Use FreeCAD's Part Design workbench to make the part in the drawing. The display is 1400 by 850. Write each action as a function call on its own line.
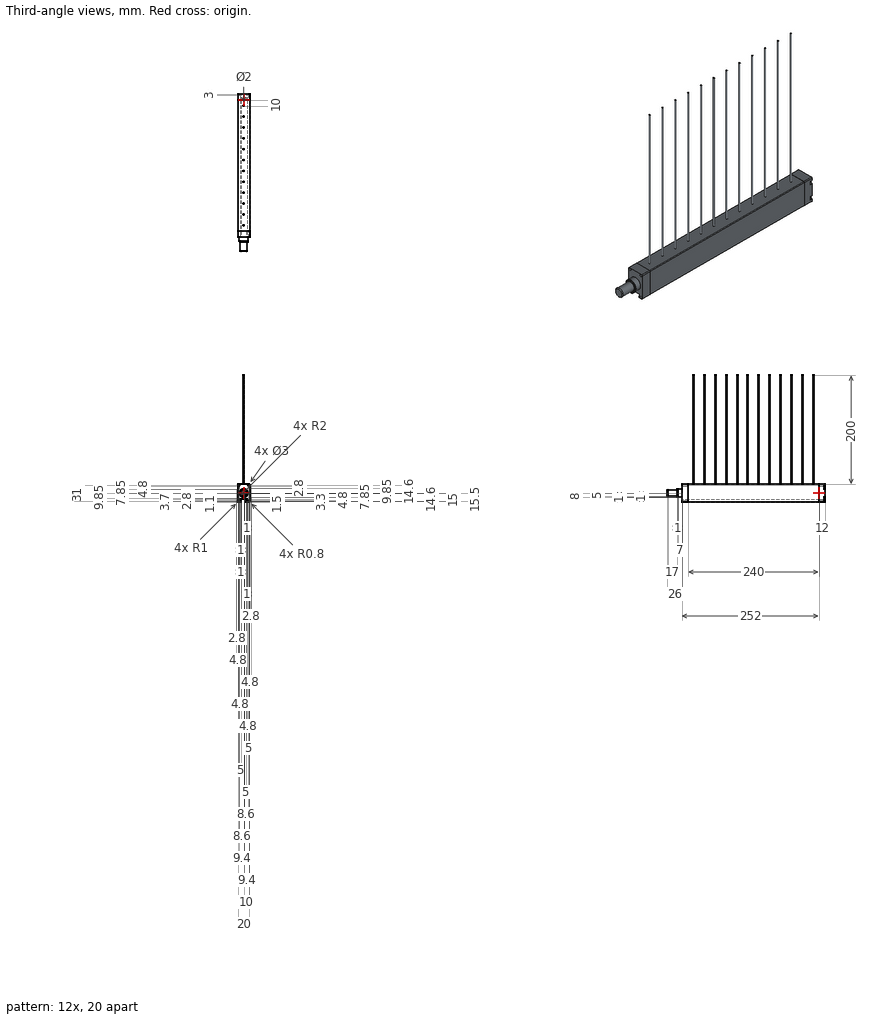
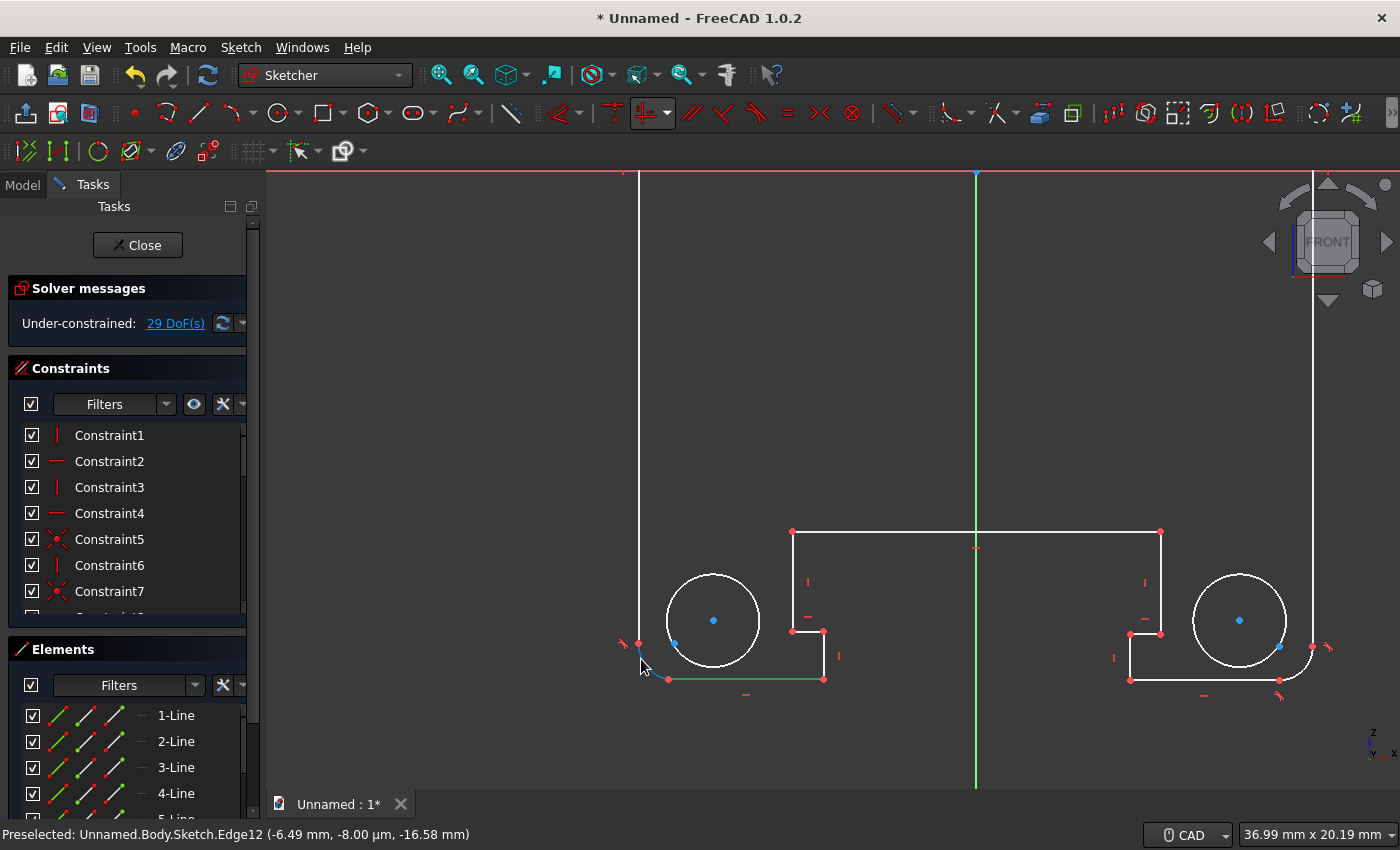
click(642, 659)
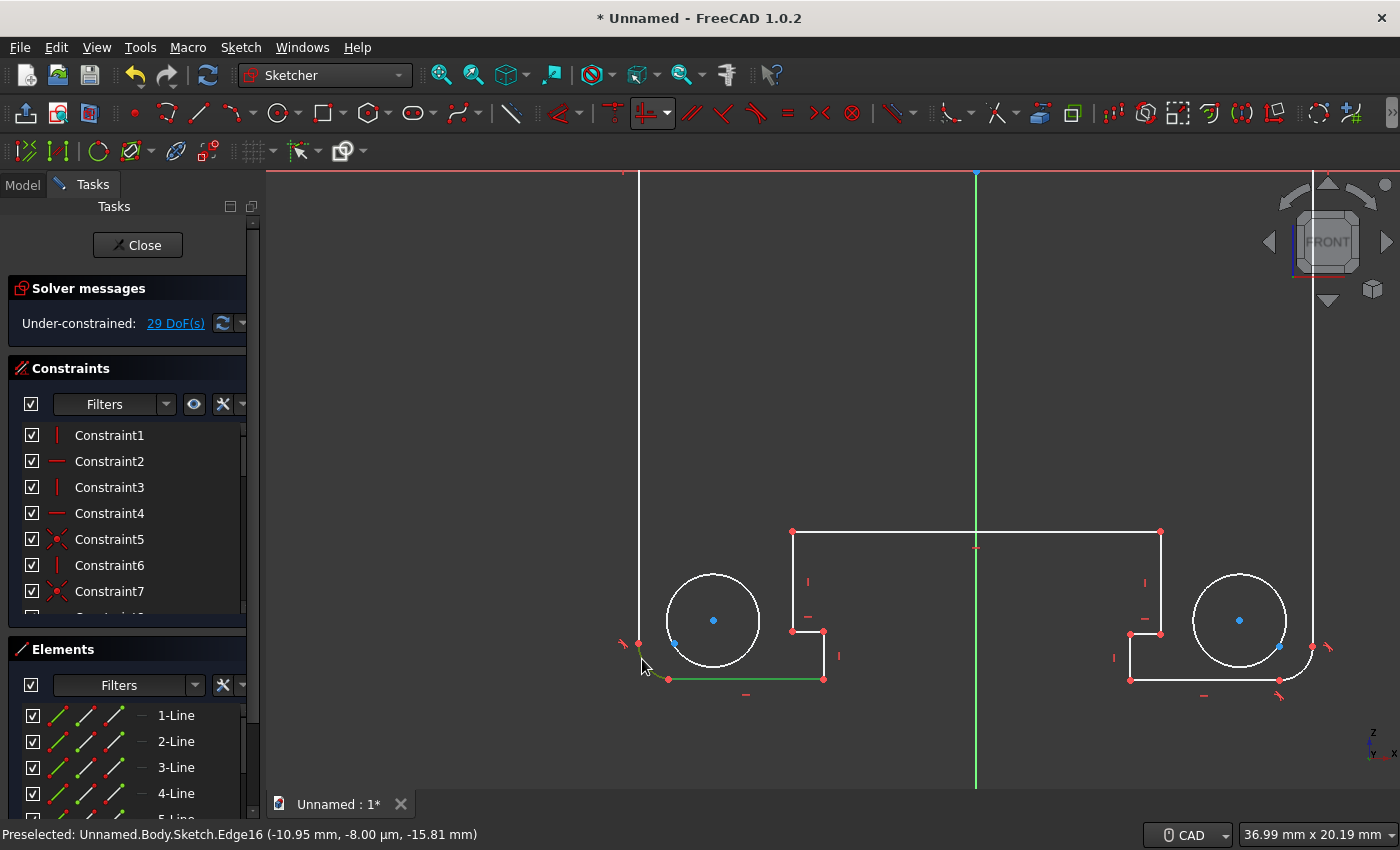
click(756, 114)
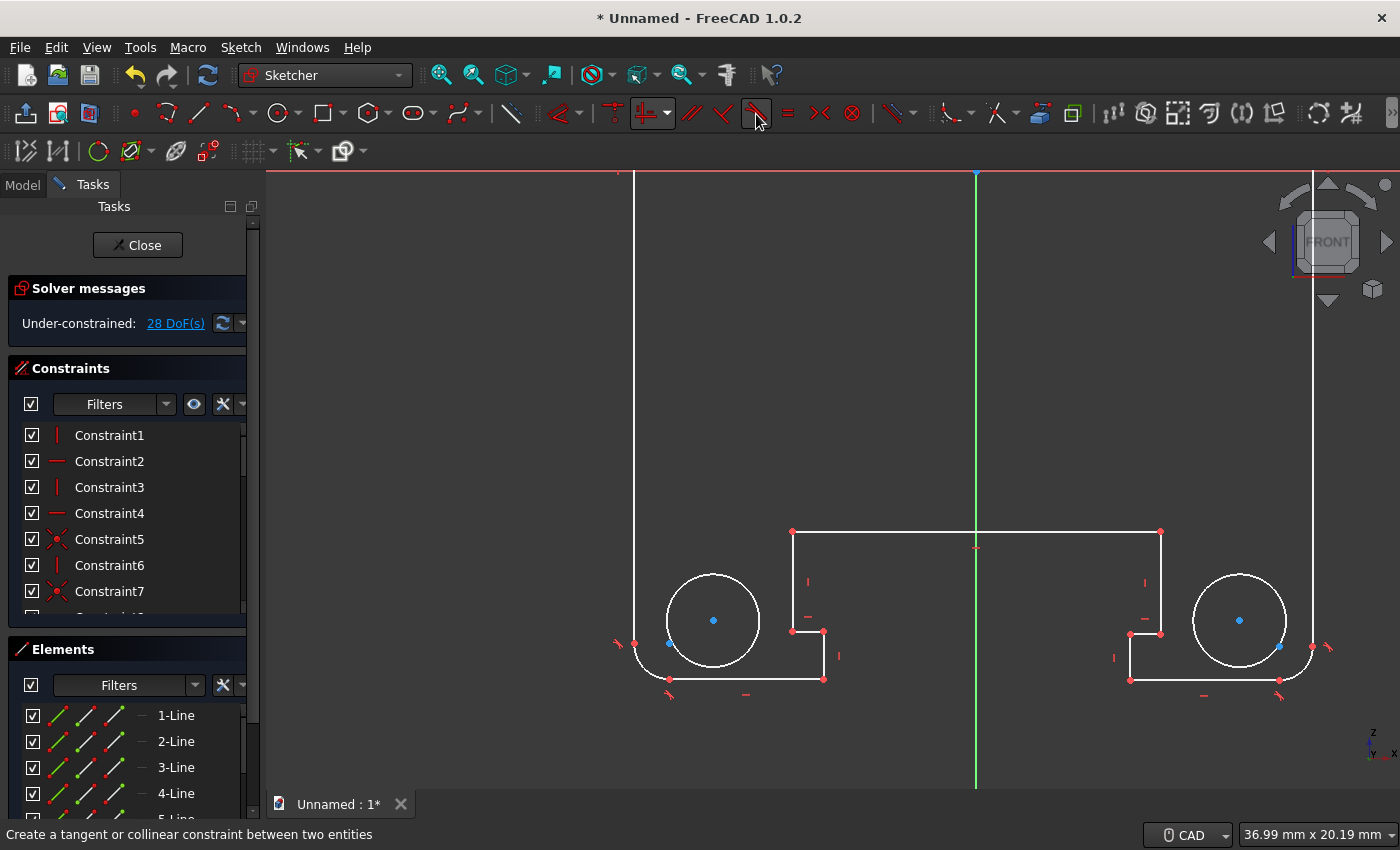
scroll(641, 659, down, 5)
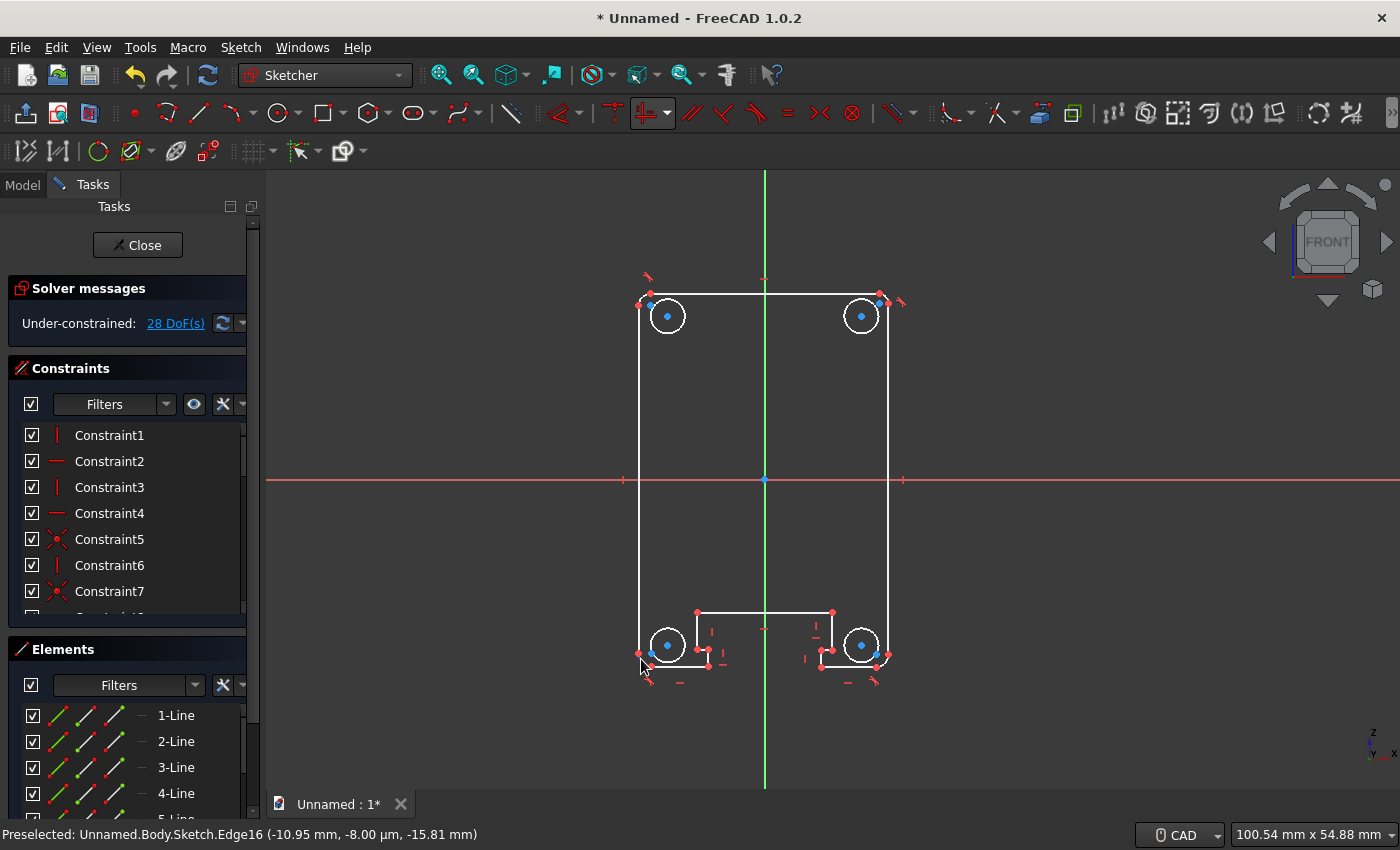
scroll(645, 295, up, 5)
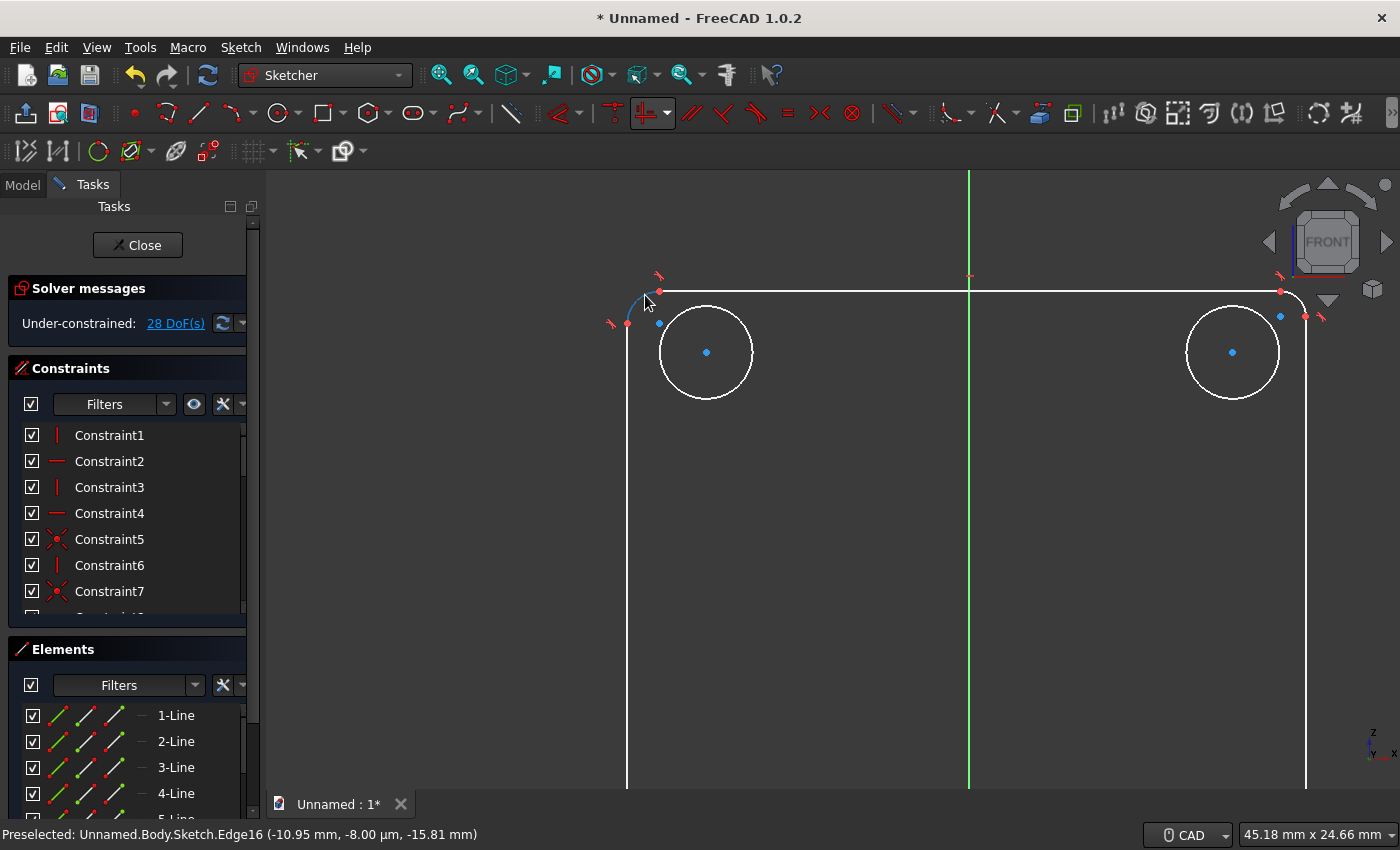
click(645, 295)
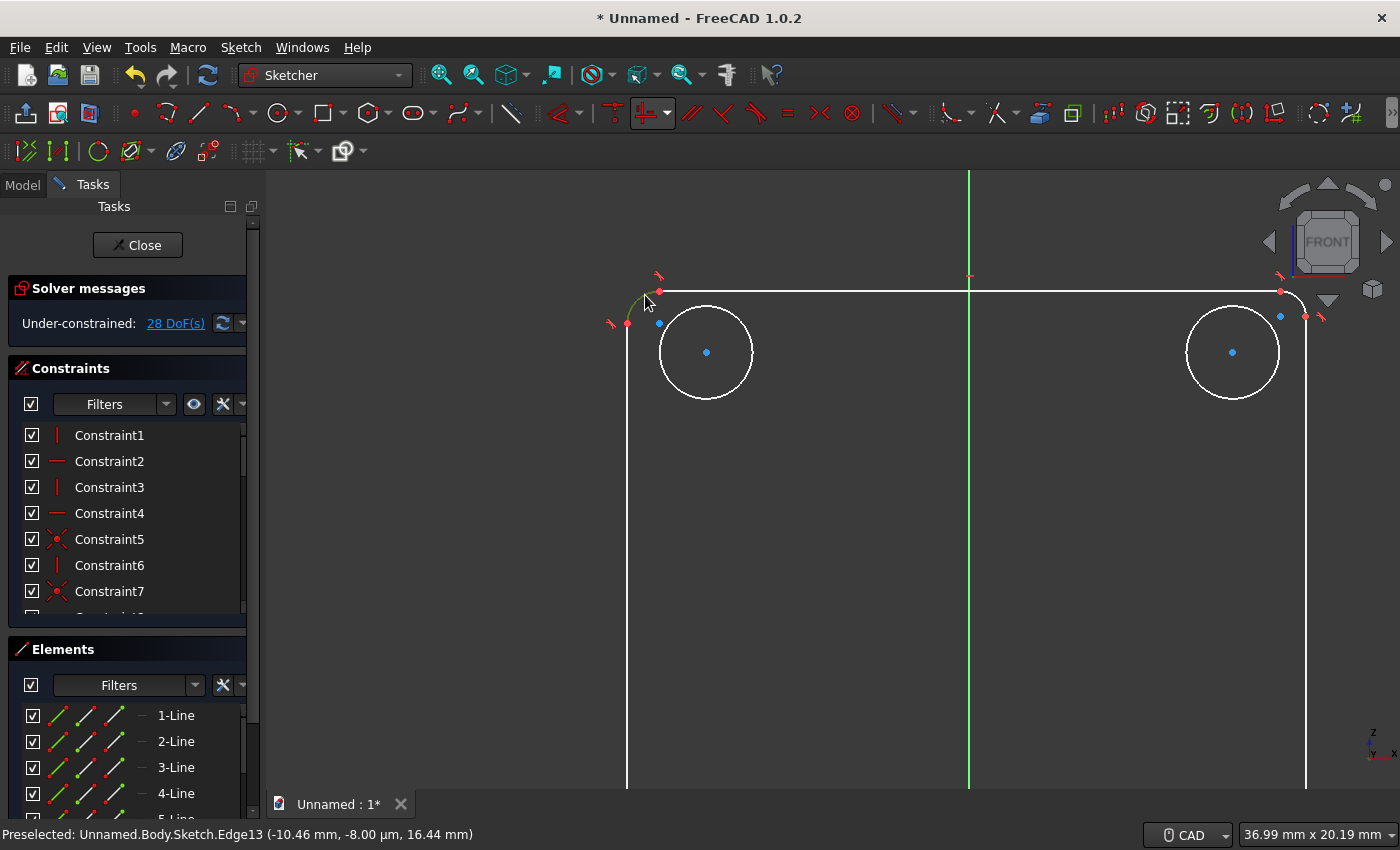
scroll(645, 294, down, 5)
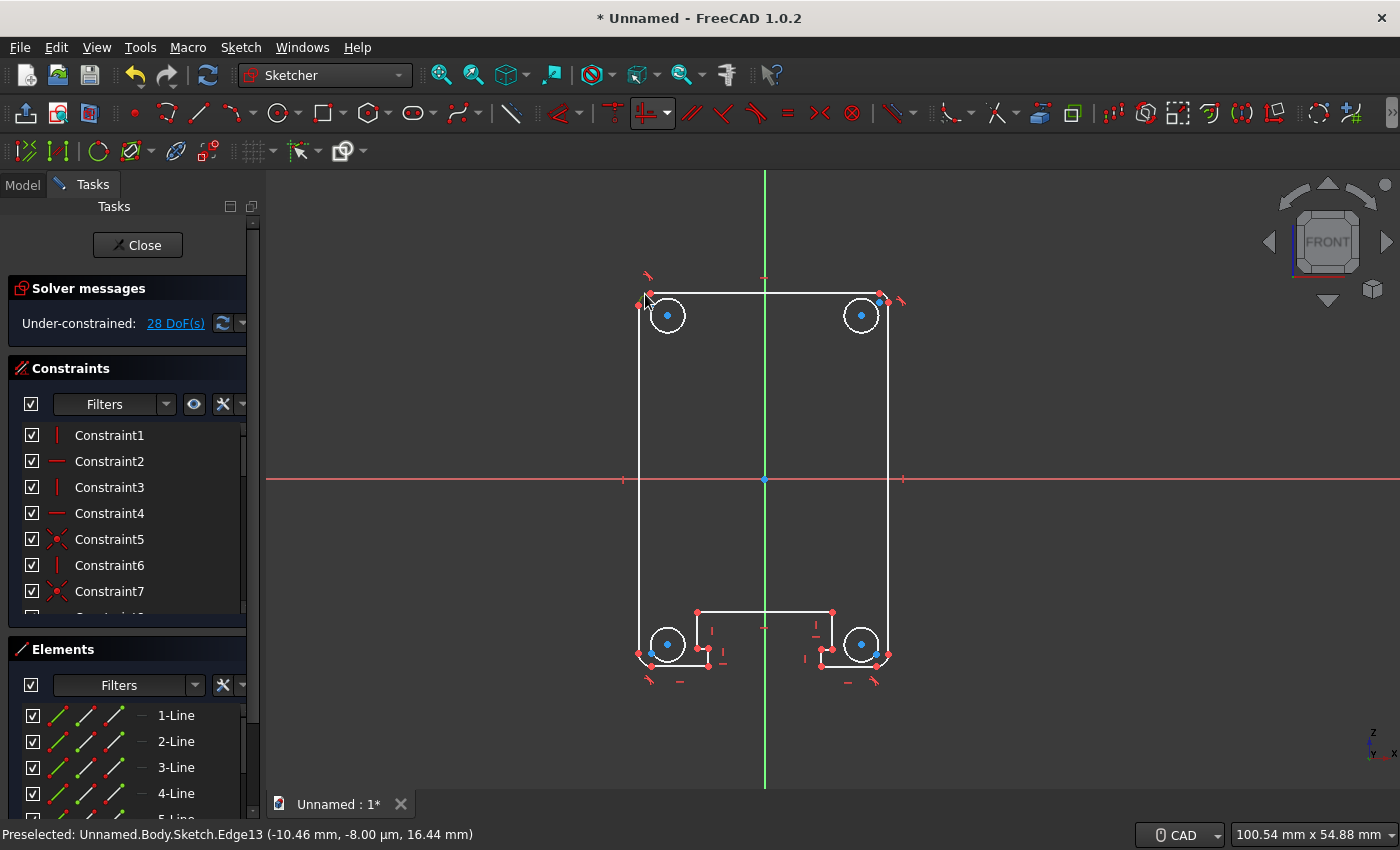
scroll(887, 298, up, 6)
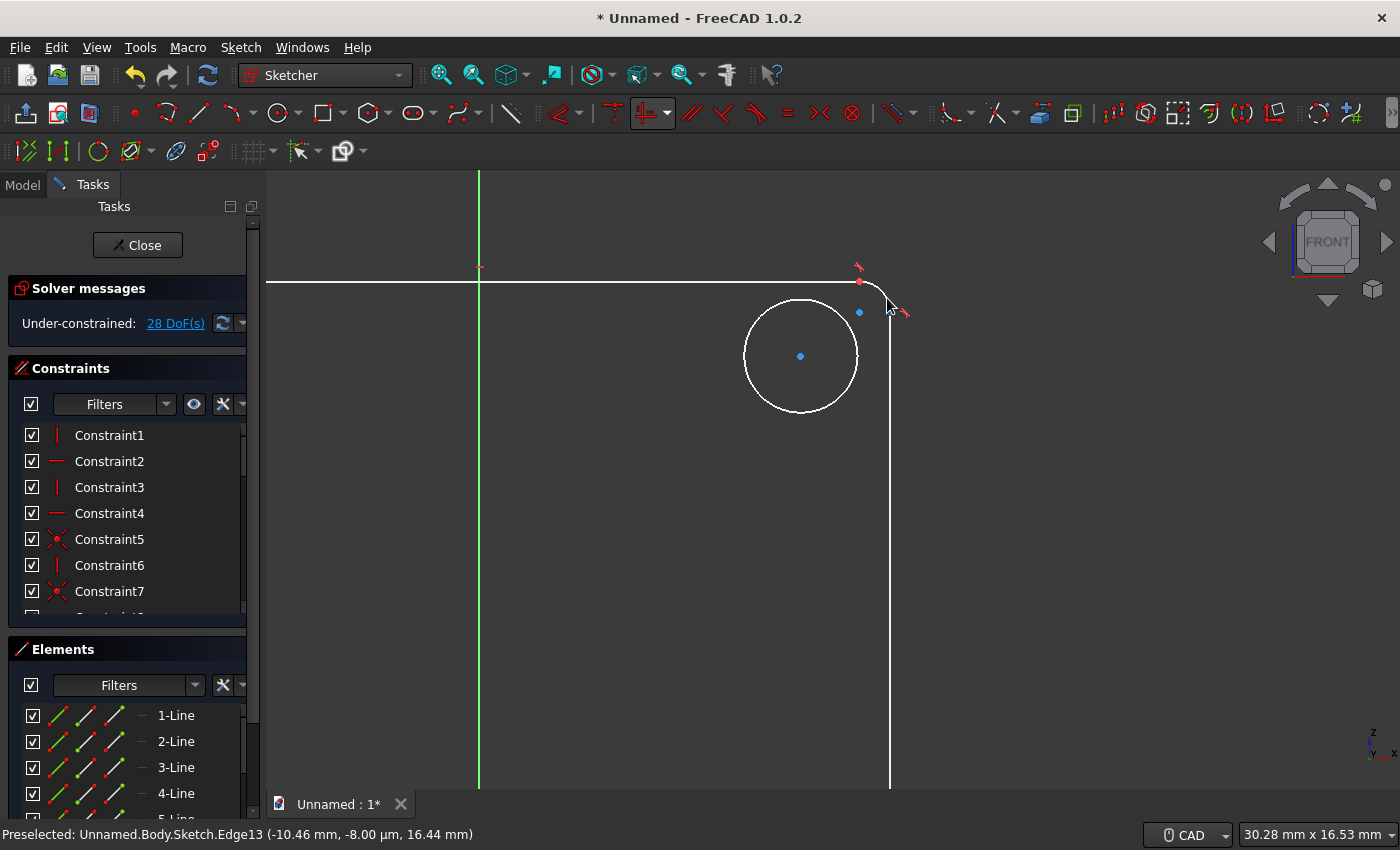
click(887, 298)